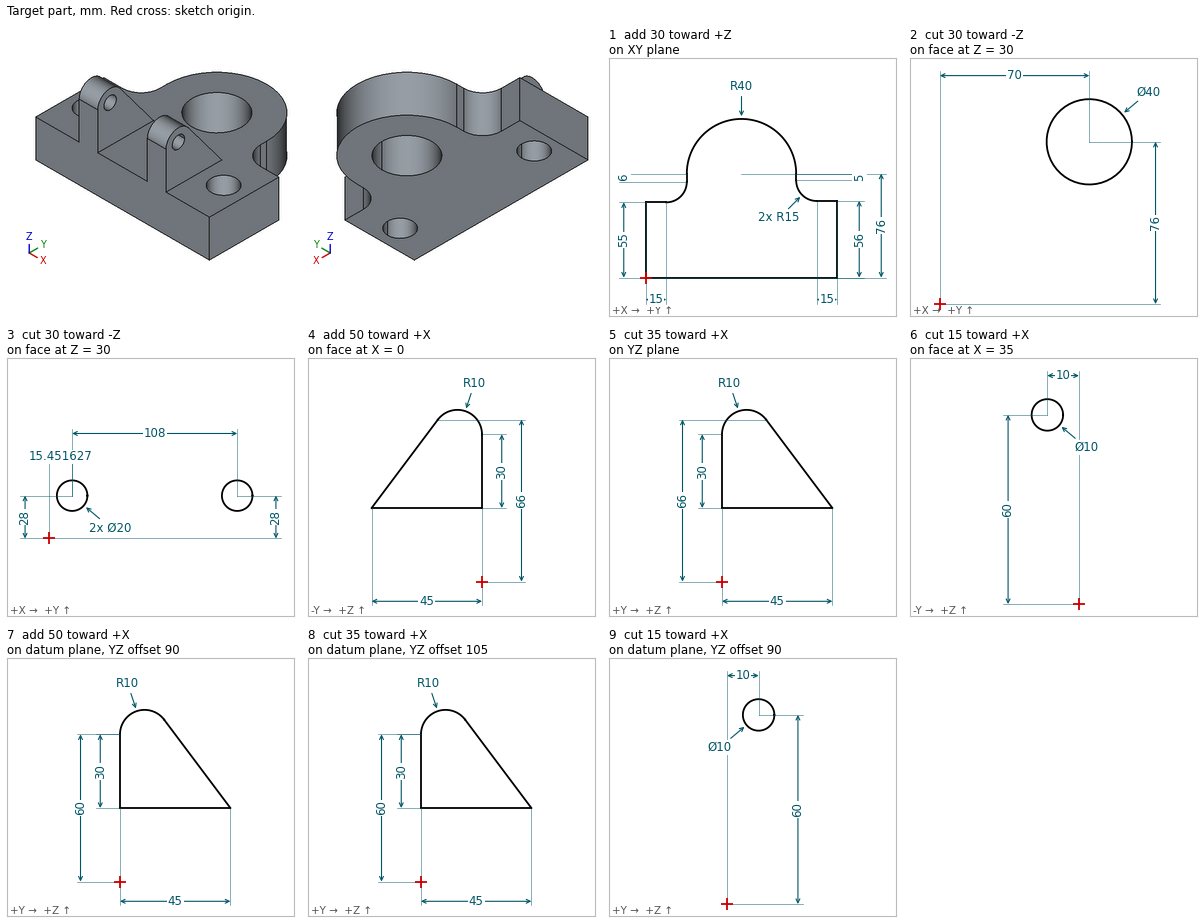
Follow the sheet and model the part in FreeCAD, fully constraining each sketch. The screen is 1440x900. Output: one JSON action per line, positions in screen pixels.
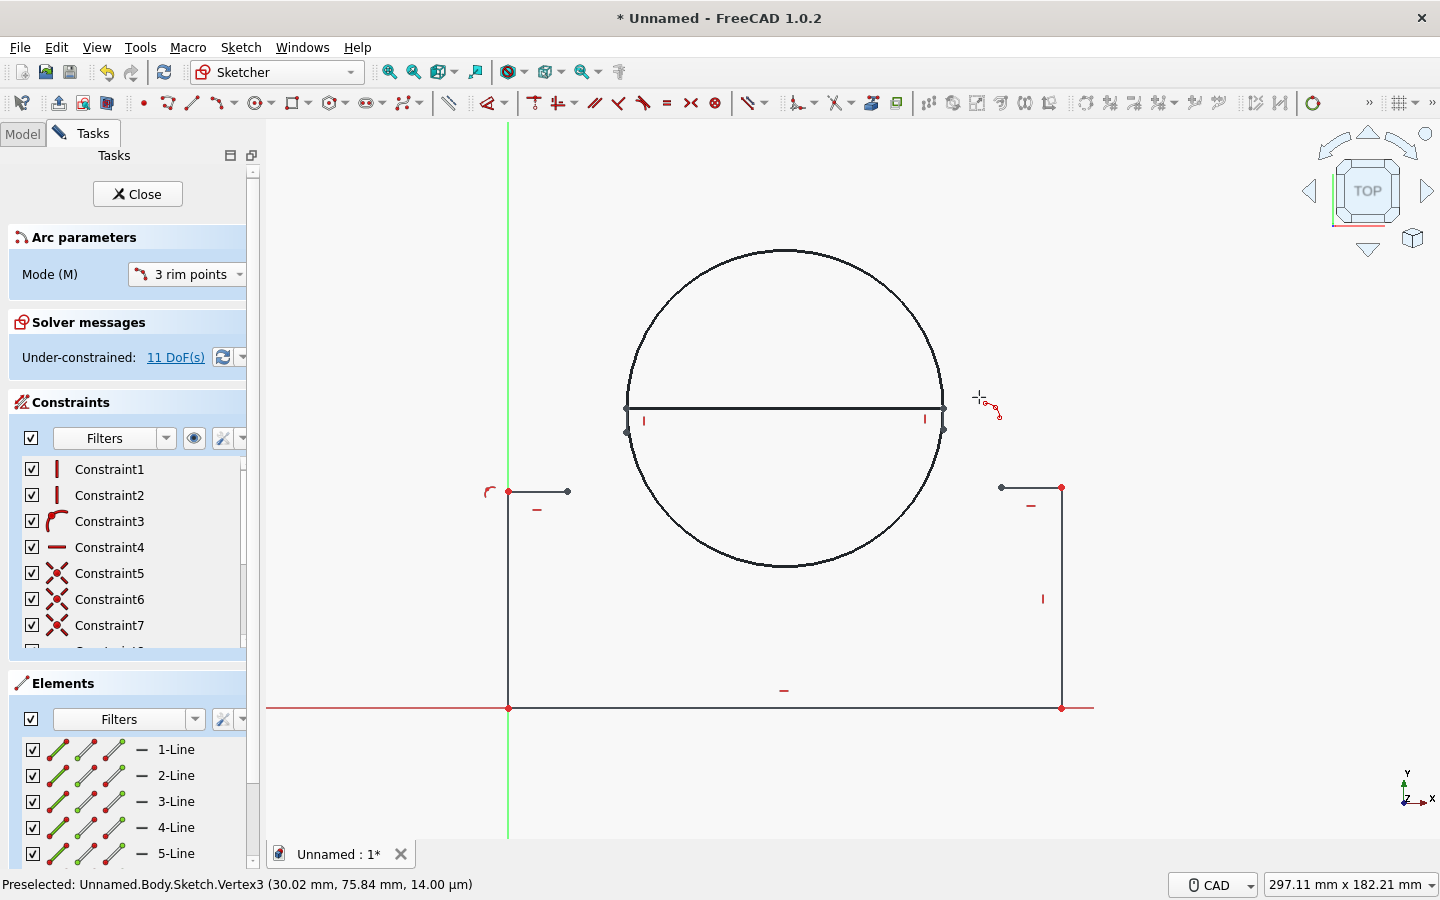
{"action": "left_click", "coordinate": [785, 250]}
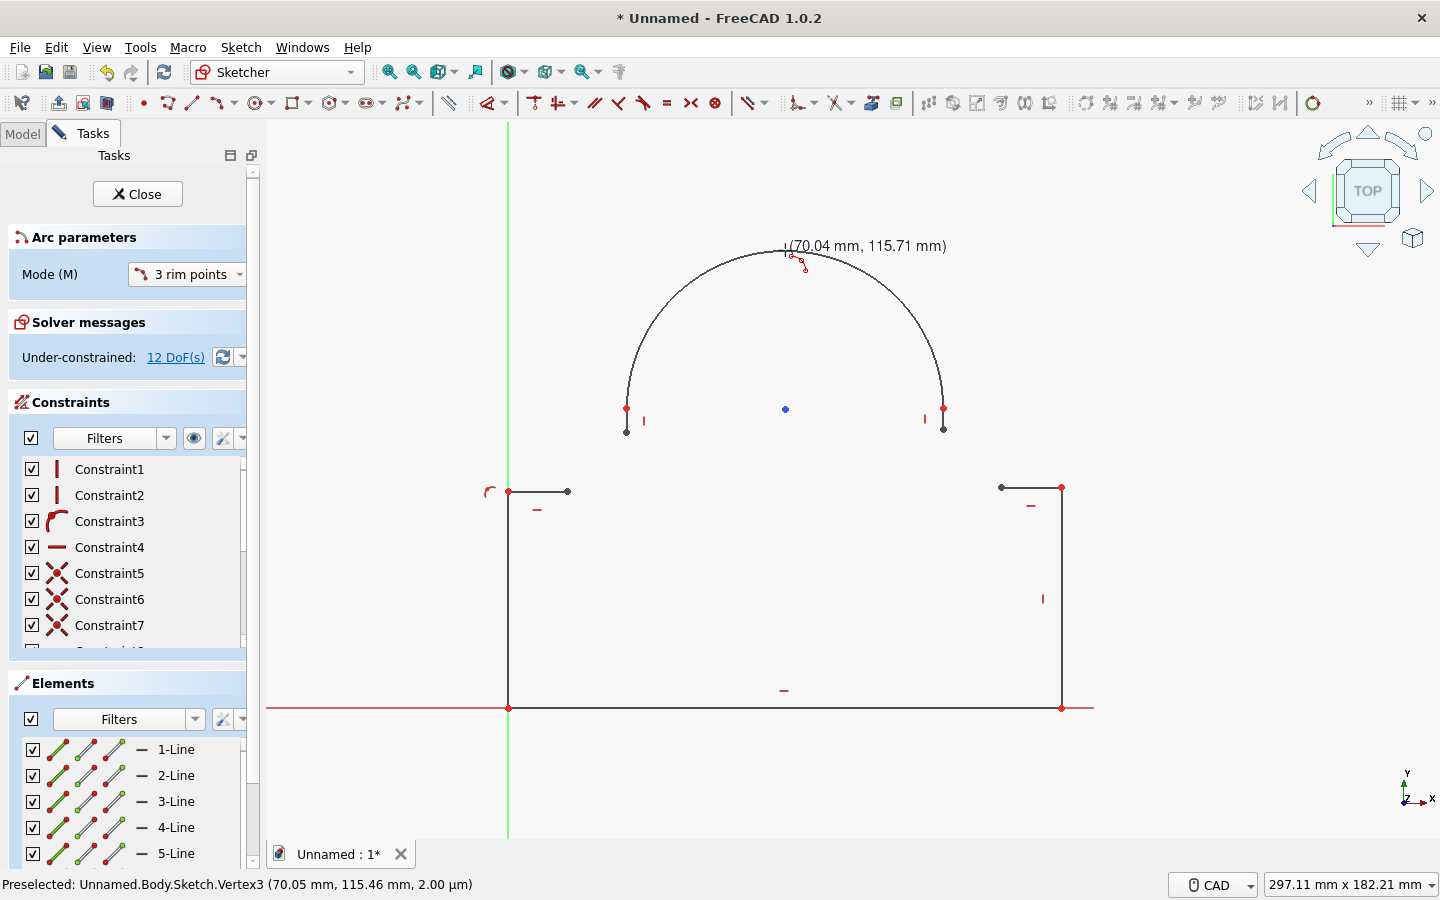
{"action": "scroll", "coordinate": [627, 432], "scroll_direction": "up", "scroll_amount": 2}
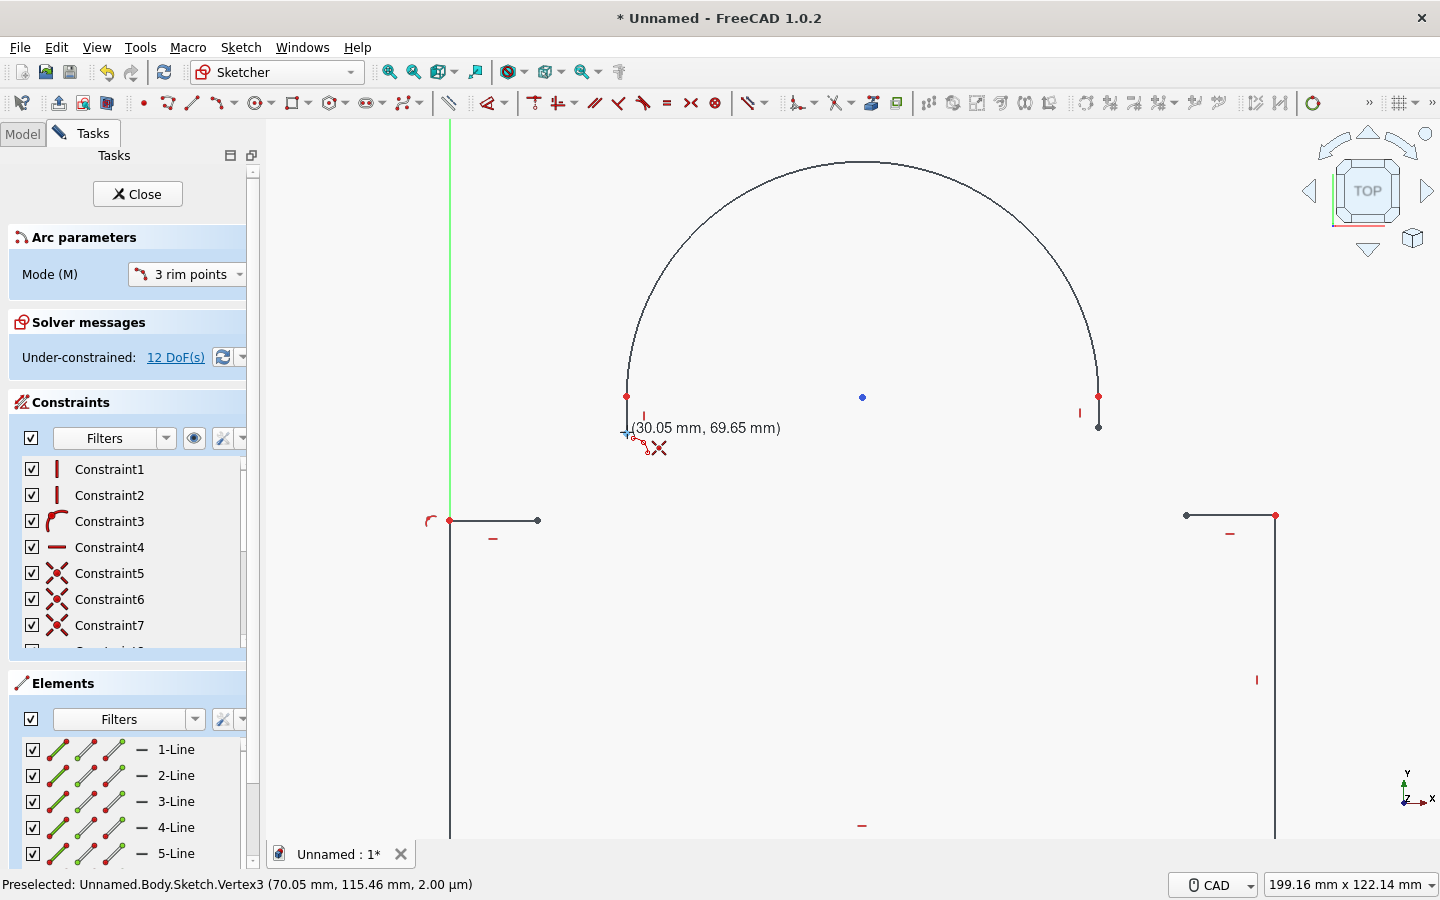
{"action": "left_click", "coordinate": [627, 433]}
{"action": "left_click", "coordinate": [537, 521]}
{"action": "left_click", "coordinate": [601, 494]}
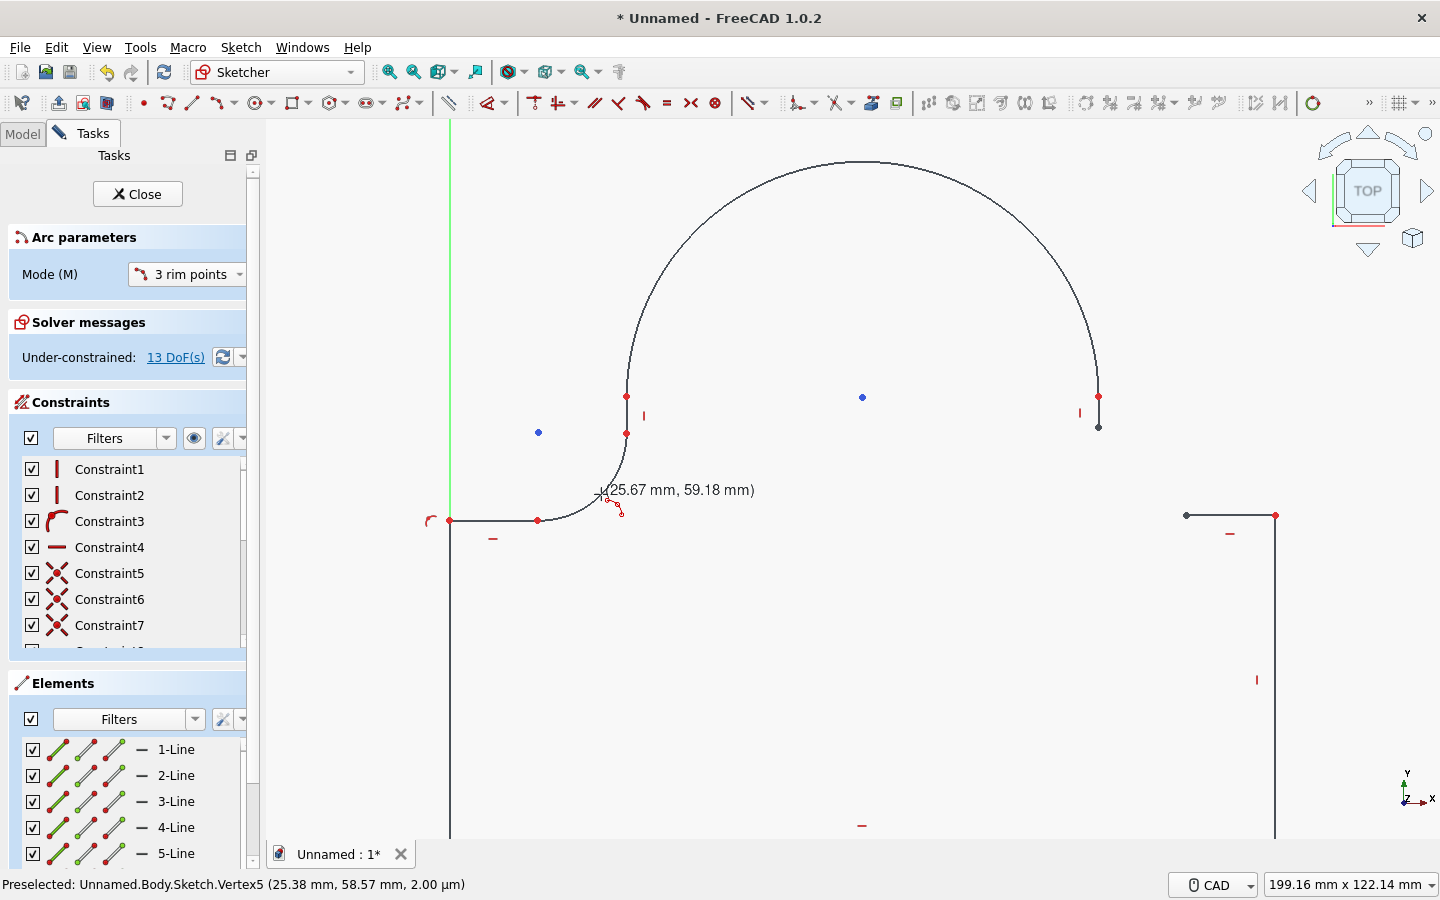
{"action": "left_click", "coordinate": [1186, 515]}
{"action": "left_click", "coordinate": [1099, 428]}
{"action": "left_click", "coordinate": [1124, 488]}
{"action": "key", "text": "Escape"}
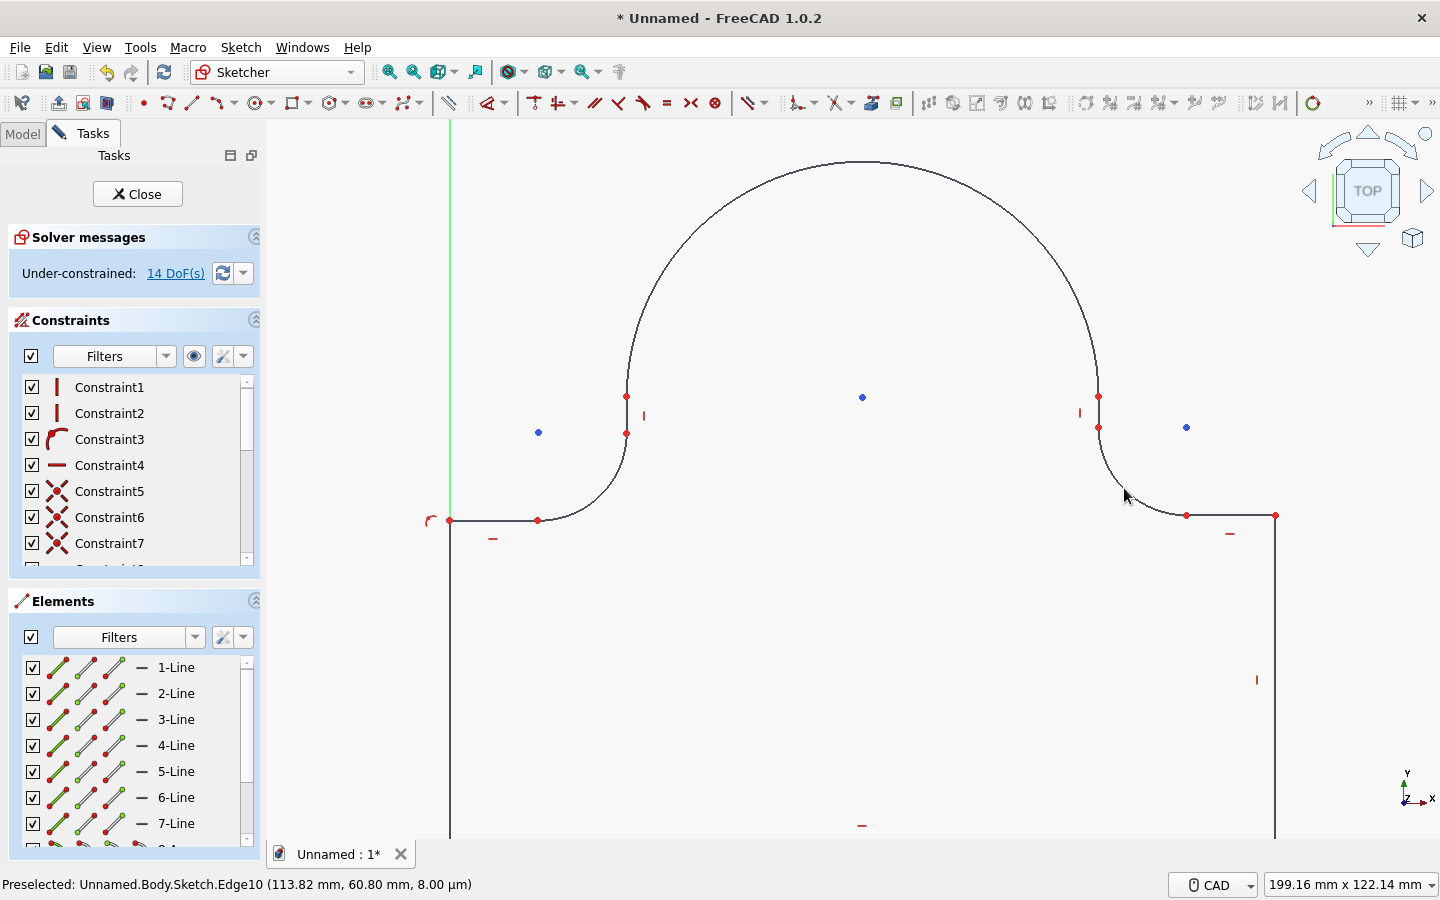
{"action": "scroll", "coordinate": [1099, 418], "scroll_direction": "up", "scroll_amount": 2}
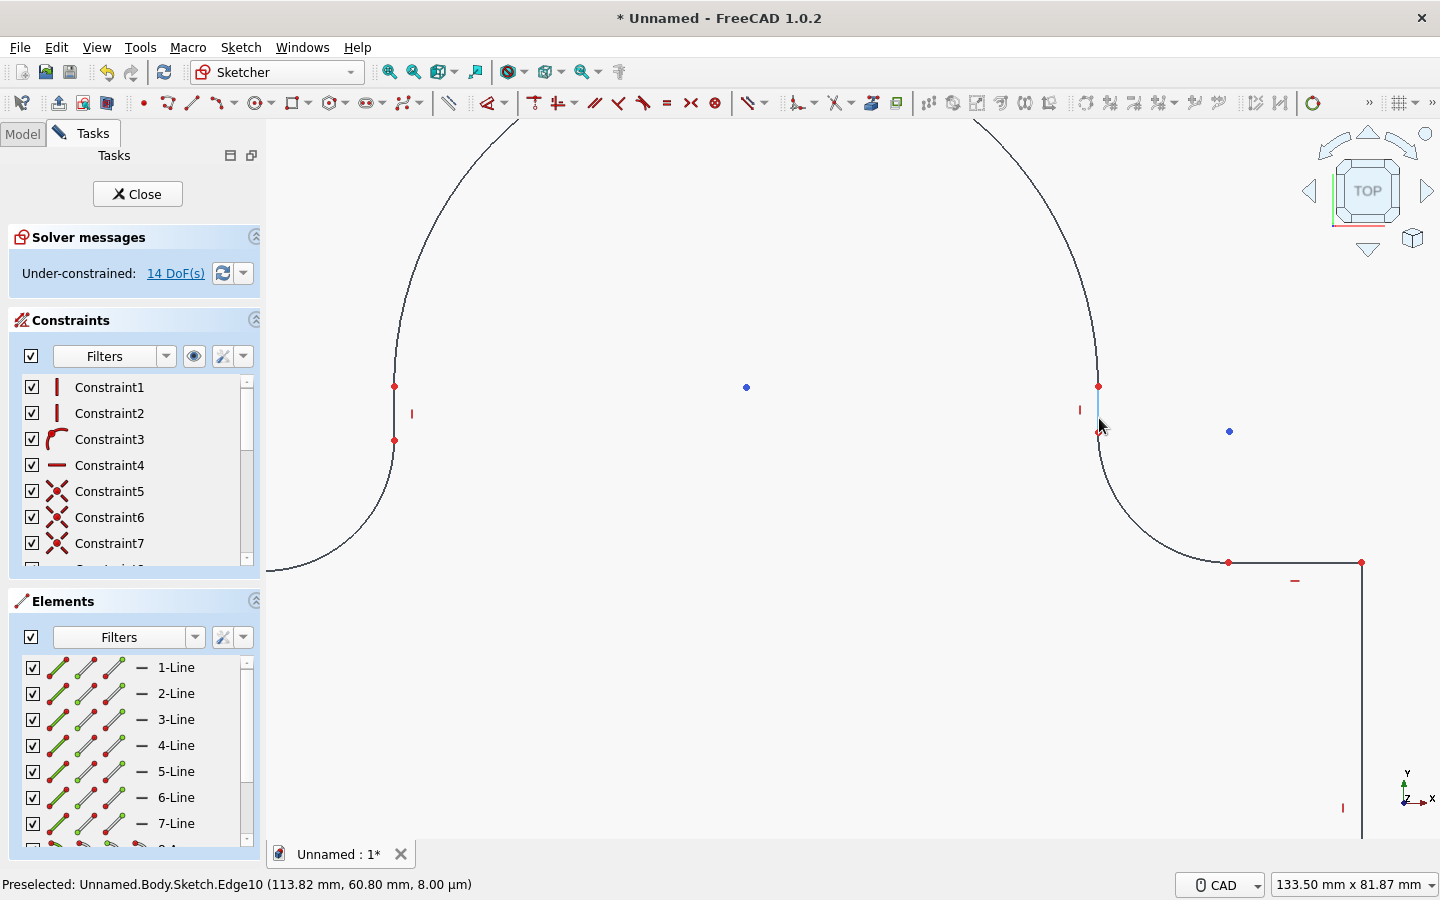
{"action": "left_click", "coordinate": [1098, 419]}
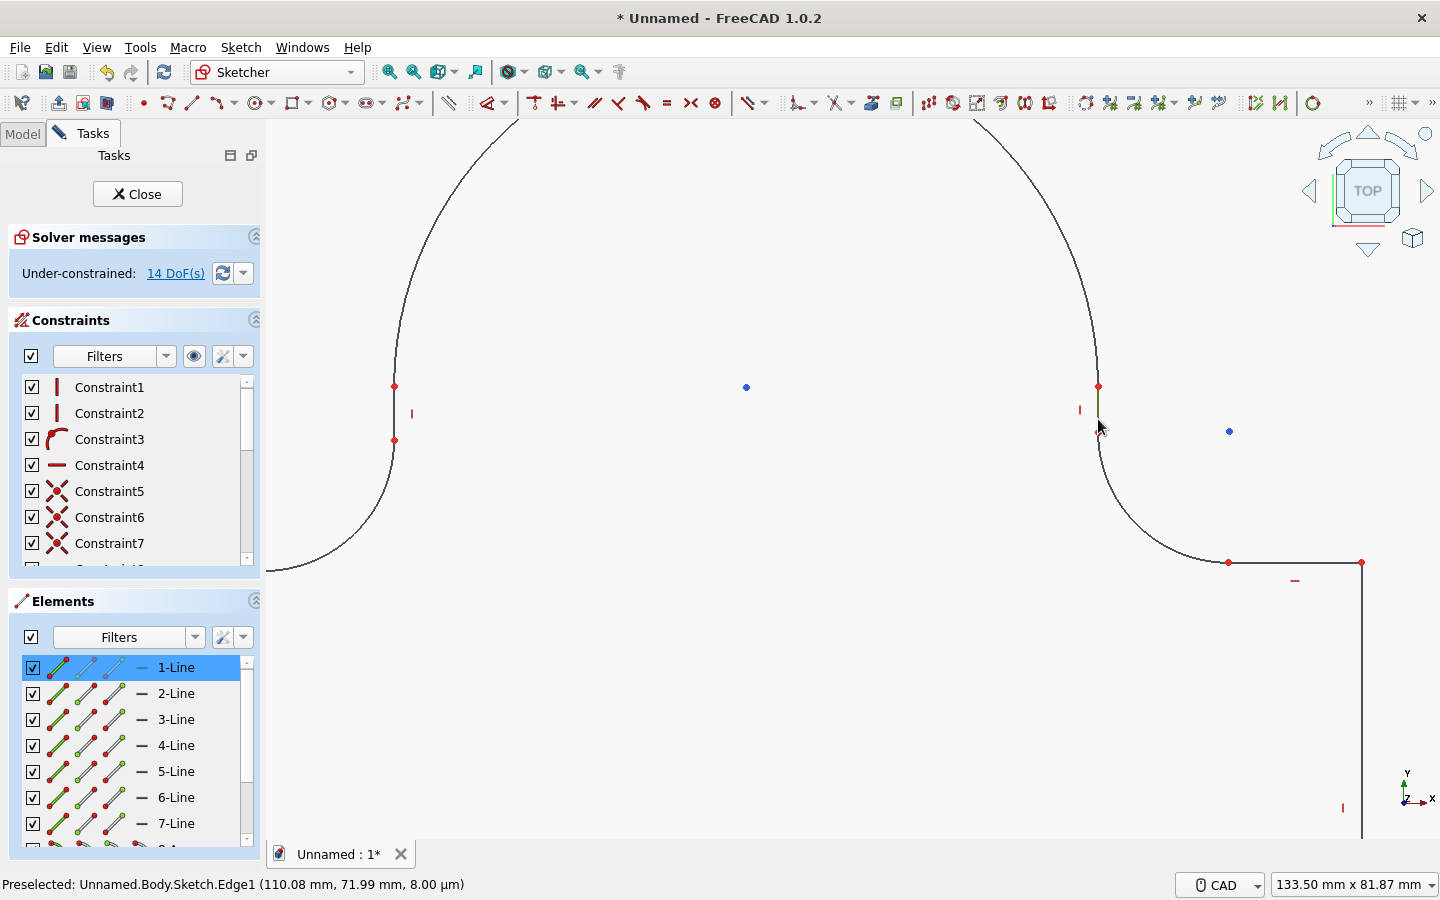
{"action": "left_click", "coordinate": [1113, 491]}